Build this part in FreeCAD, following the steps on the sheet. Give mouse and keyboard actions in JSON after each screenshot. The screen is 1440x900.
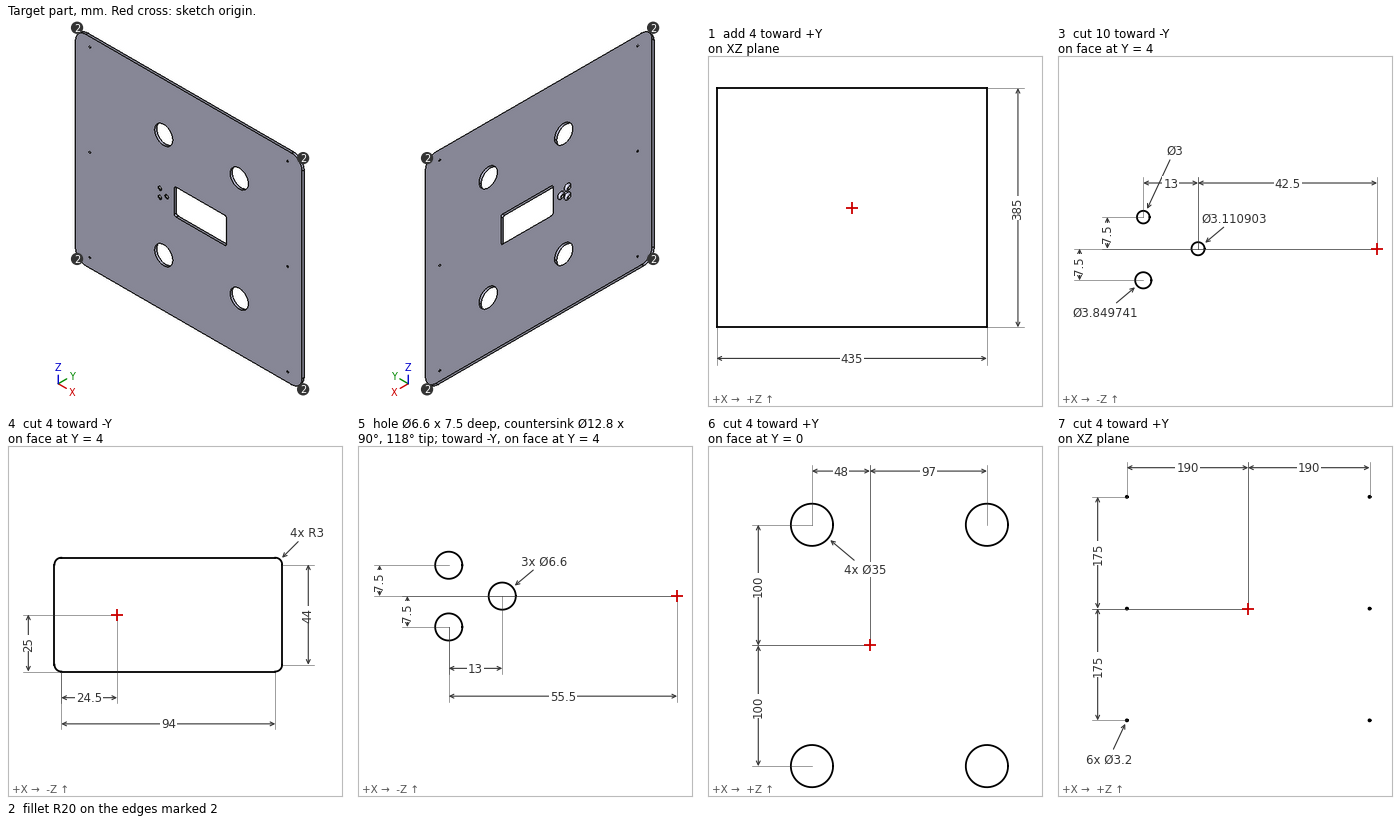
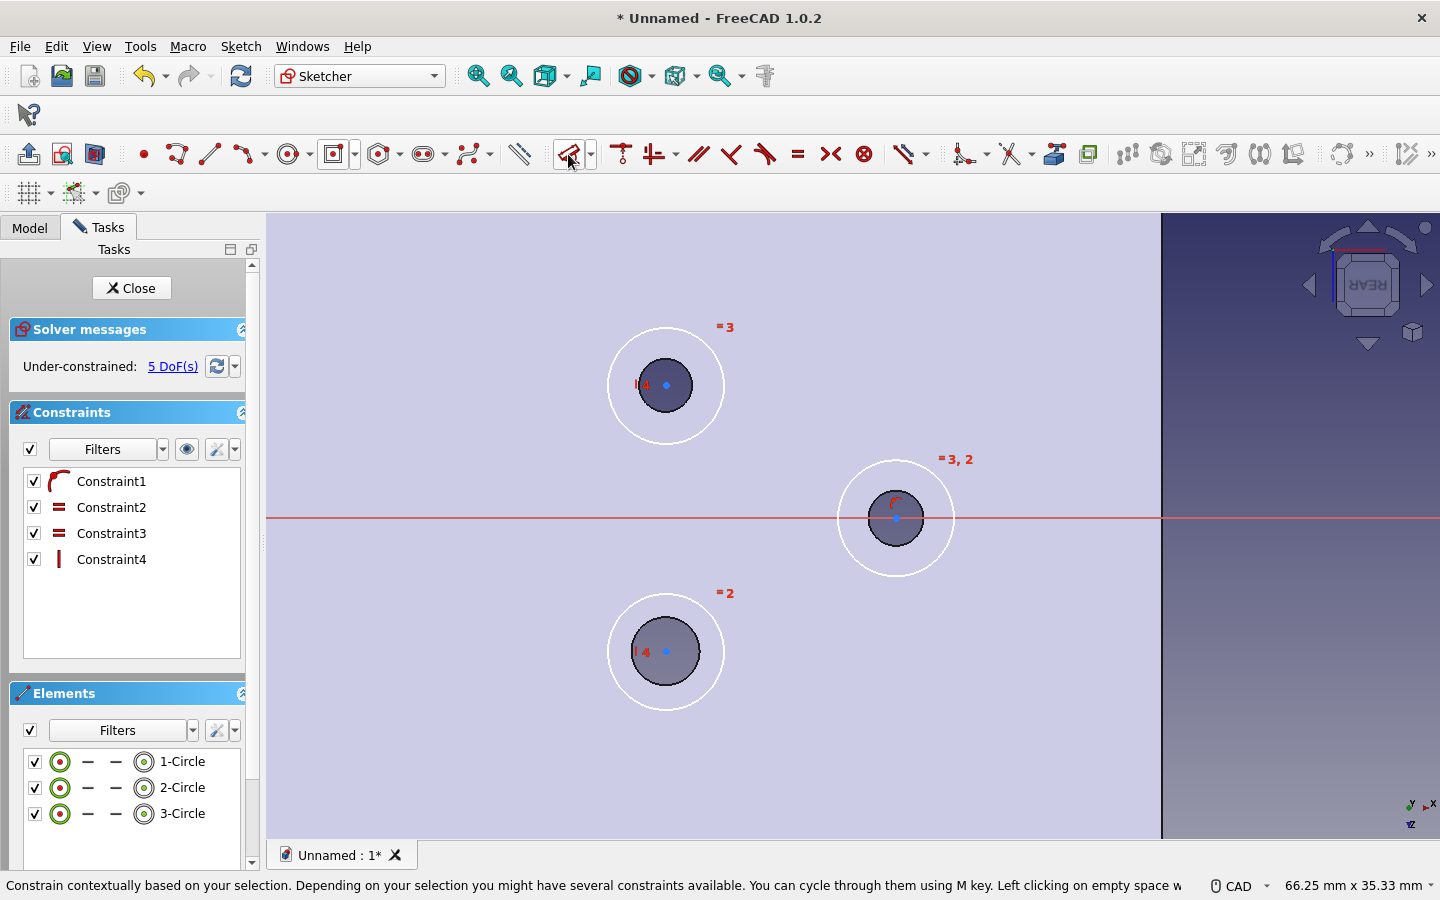
{"action": "left_click", "coordinate": [707, 611]}
{"action": "left_click", "coordinate": [730, 588]}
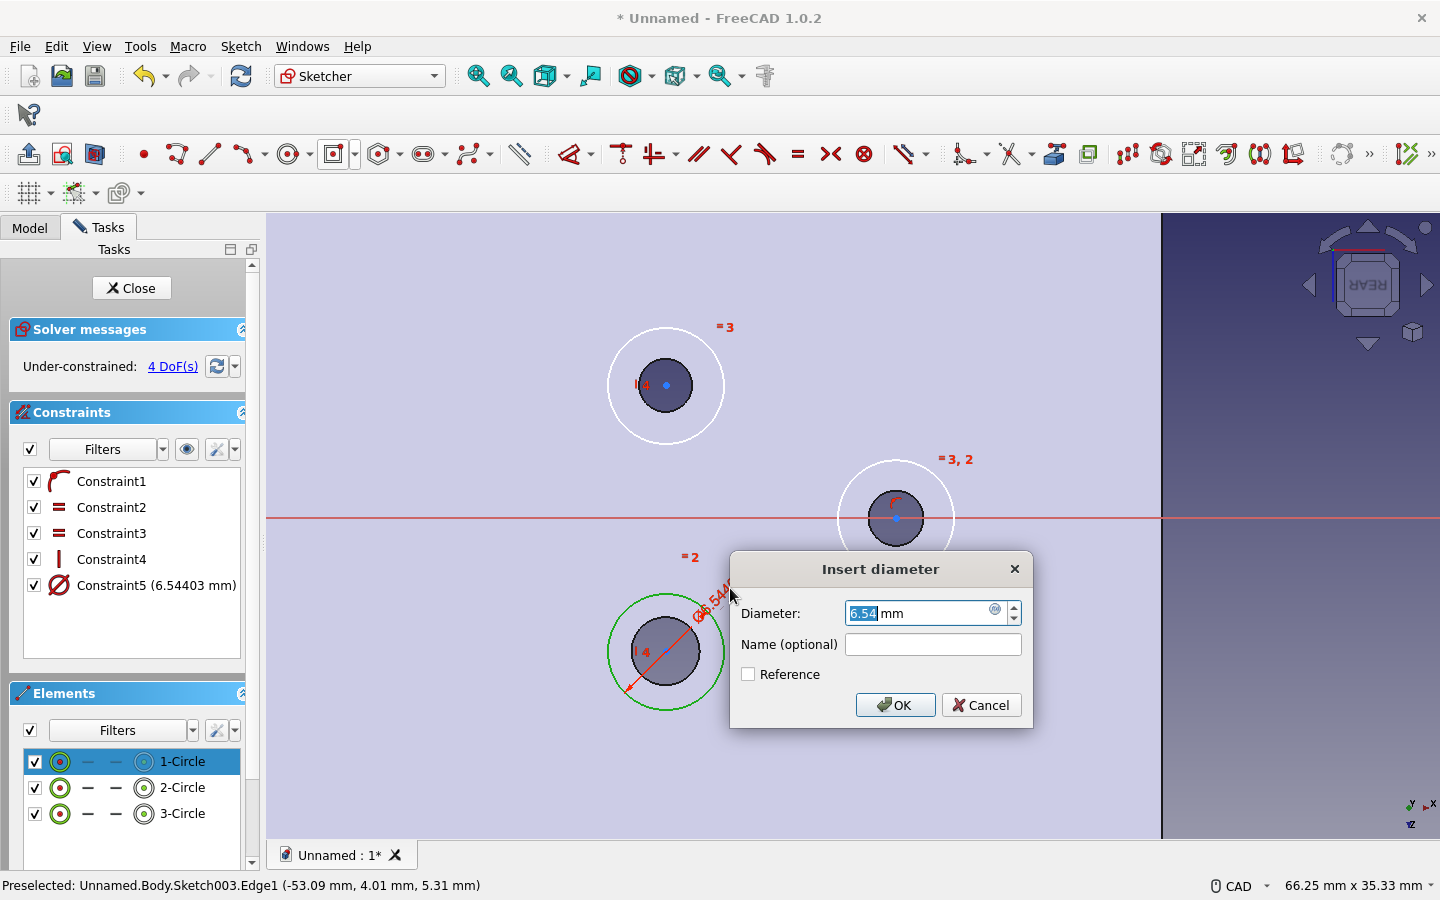
{"action": "type", "text": "6.6"}
{"action": "key", "text": "Return"}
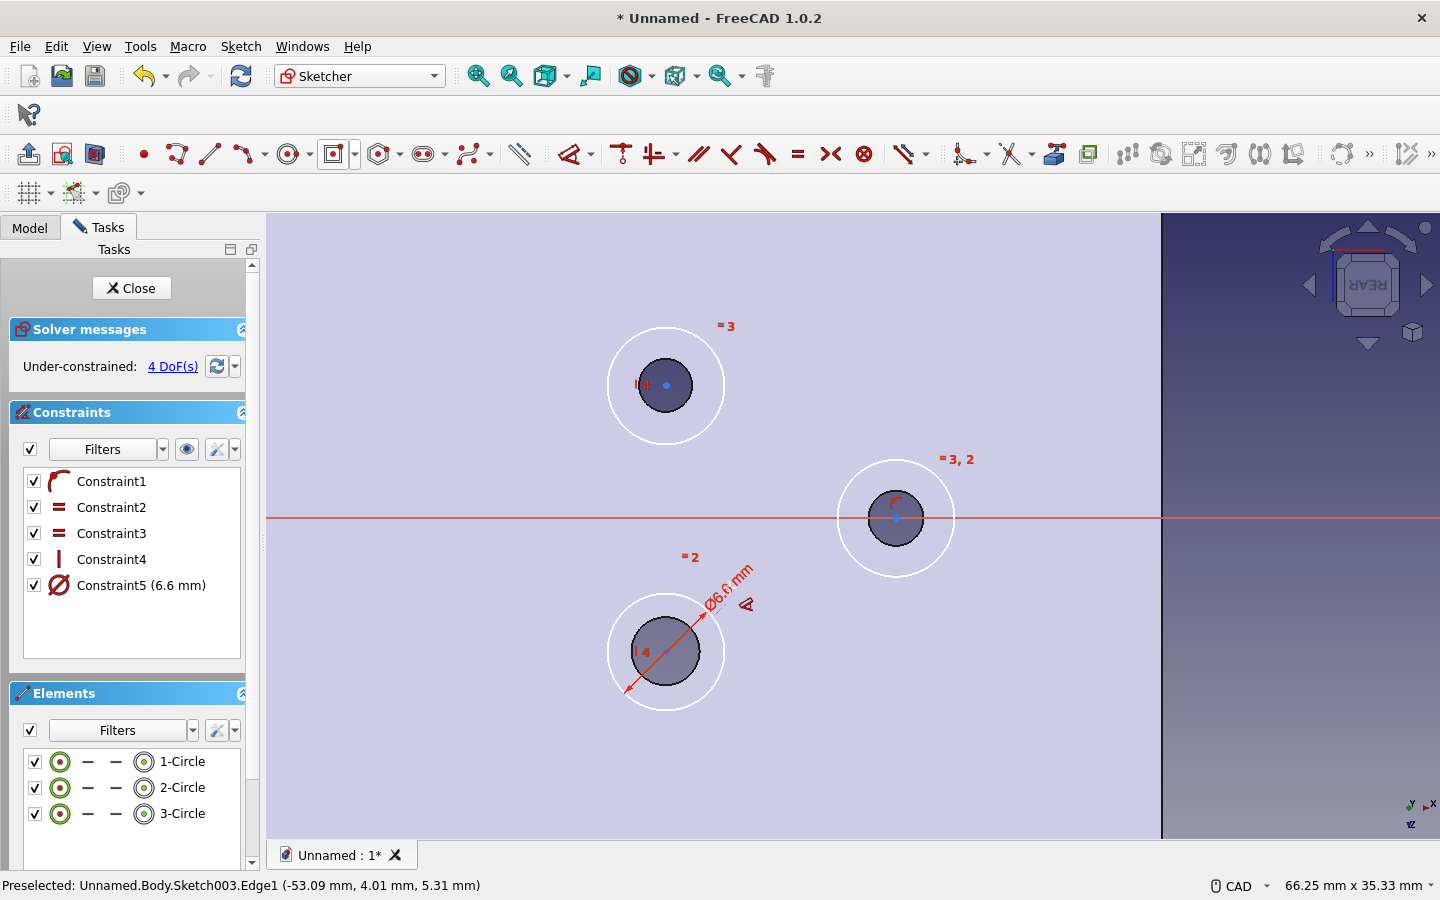
{"action": "left_click", "coordinate": [666, 652]}
{"action": "left_click", "coordinate": [632, 585]}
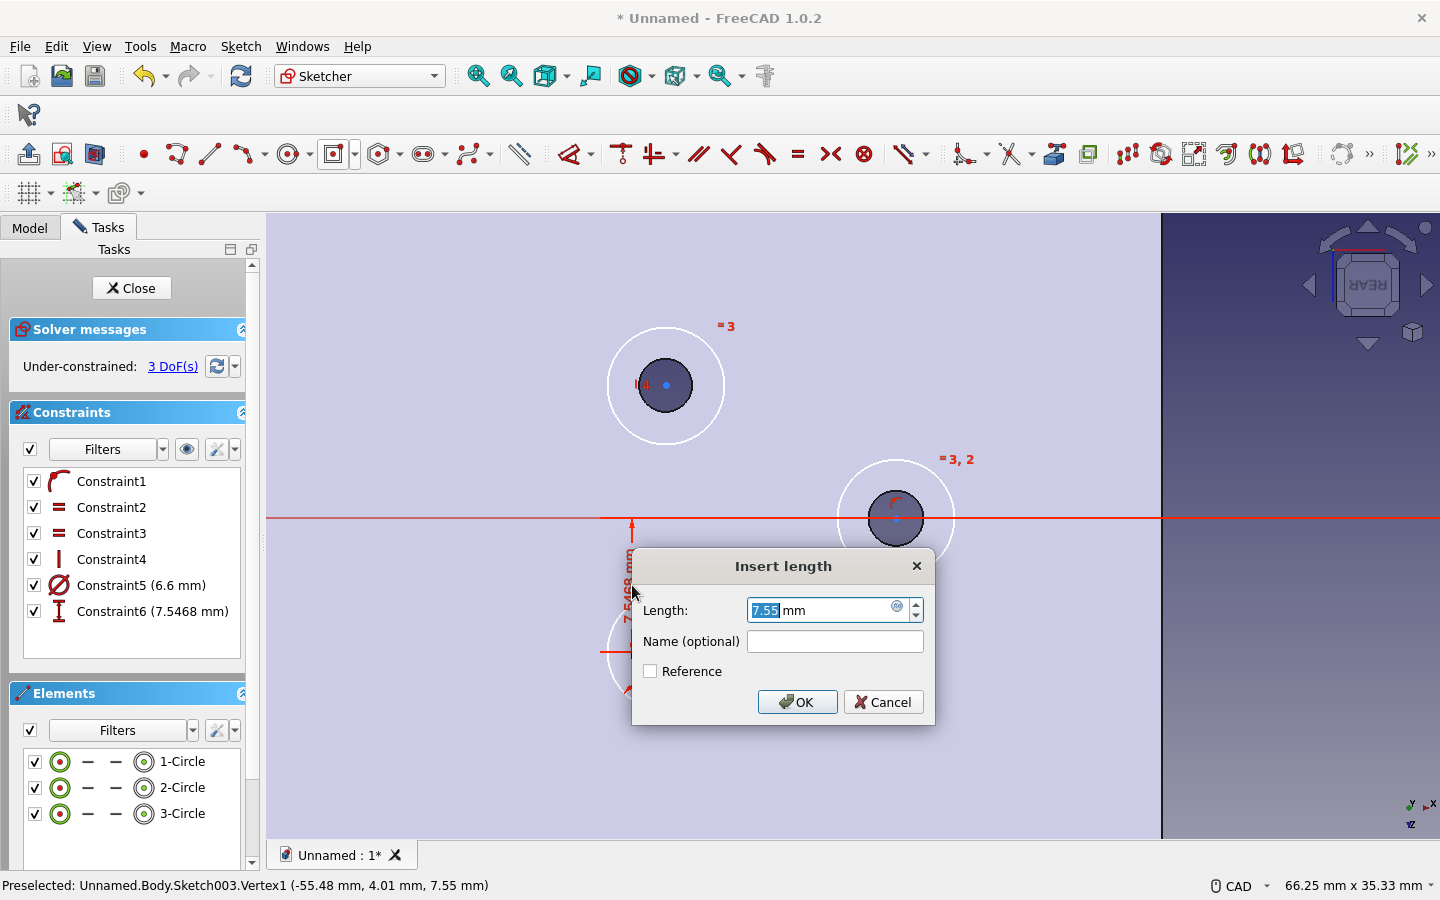
{"action": "type", "text": "7.5"}
{"action": "key", "text": "Return"}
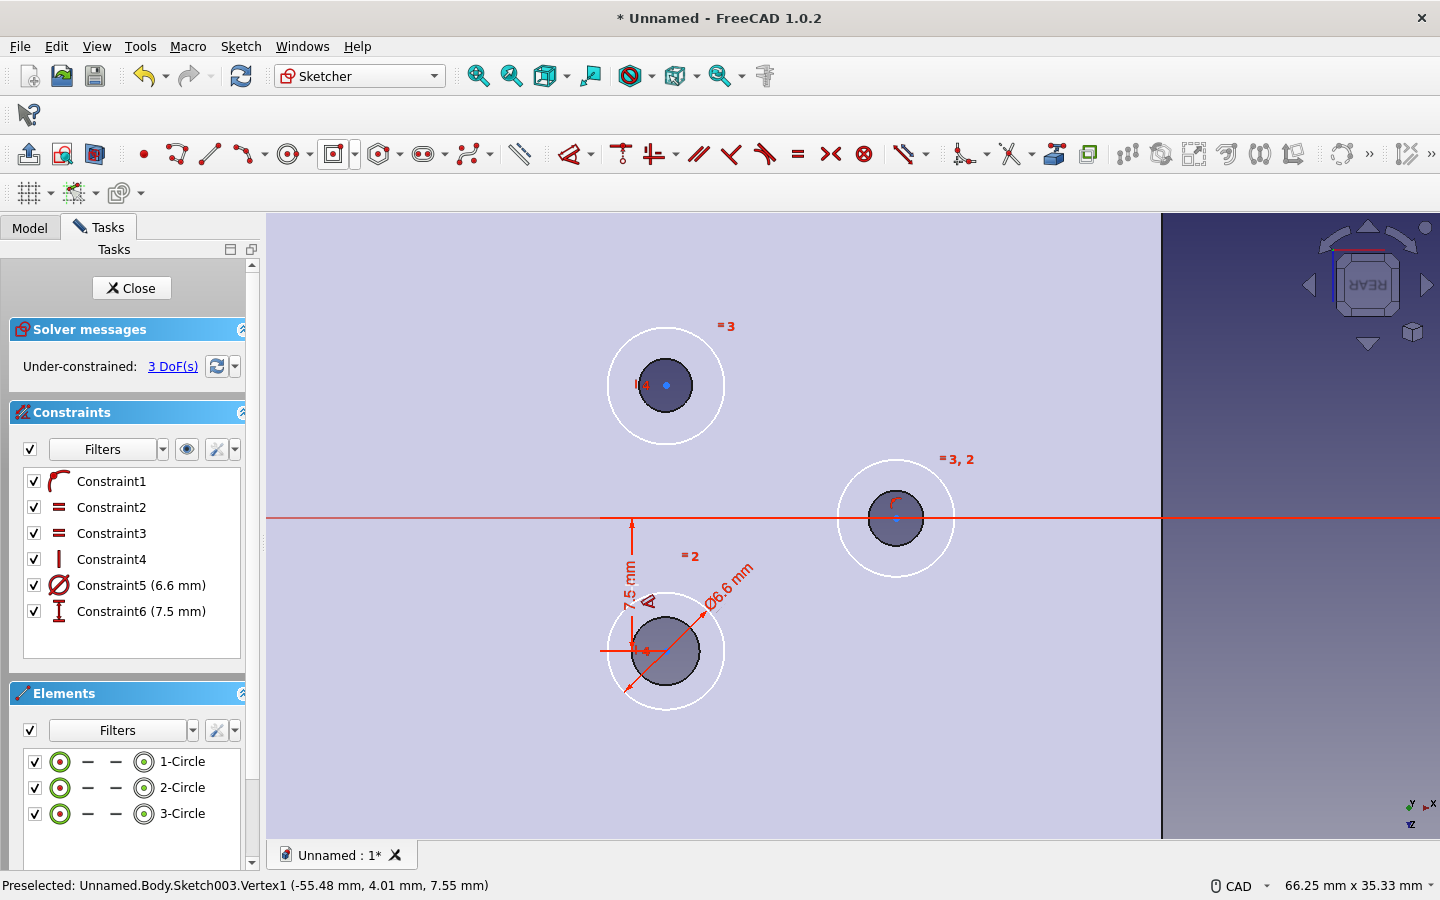
{"action": "left_click", "coordinate": [666, 386]}
{"action": "left_click", "coordinate": [632, 452]}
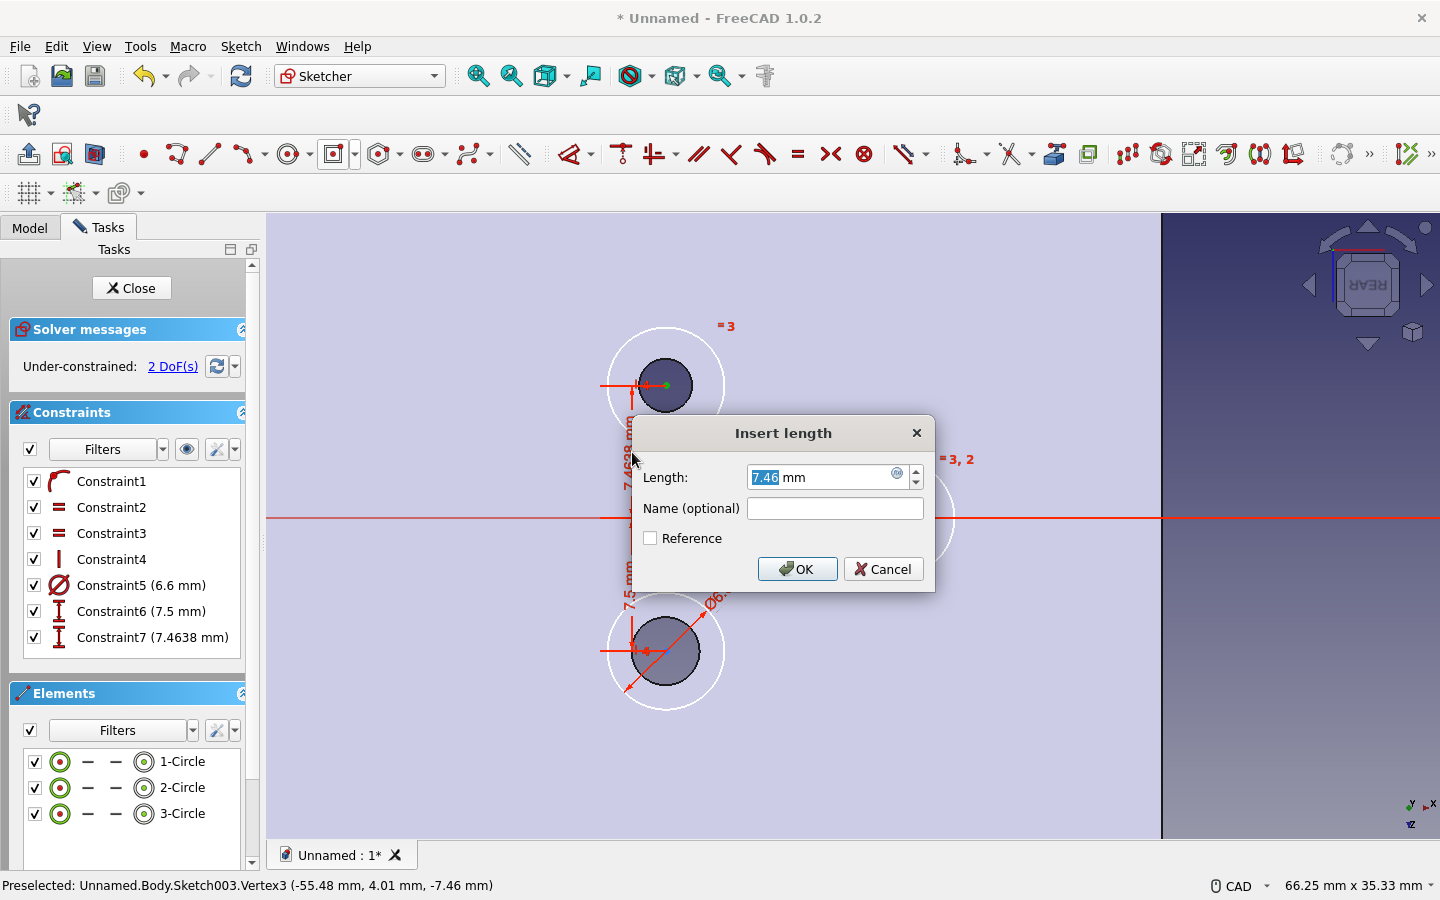
{"action": "type", "text": "7.5"}
{"action": "key", "text": "Return"}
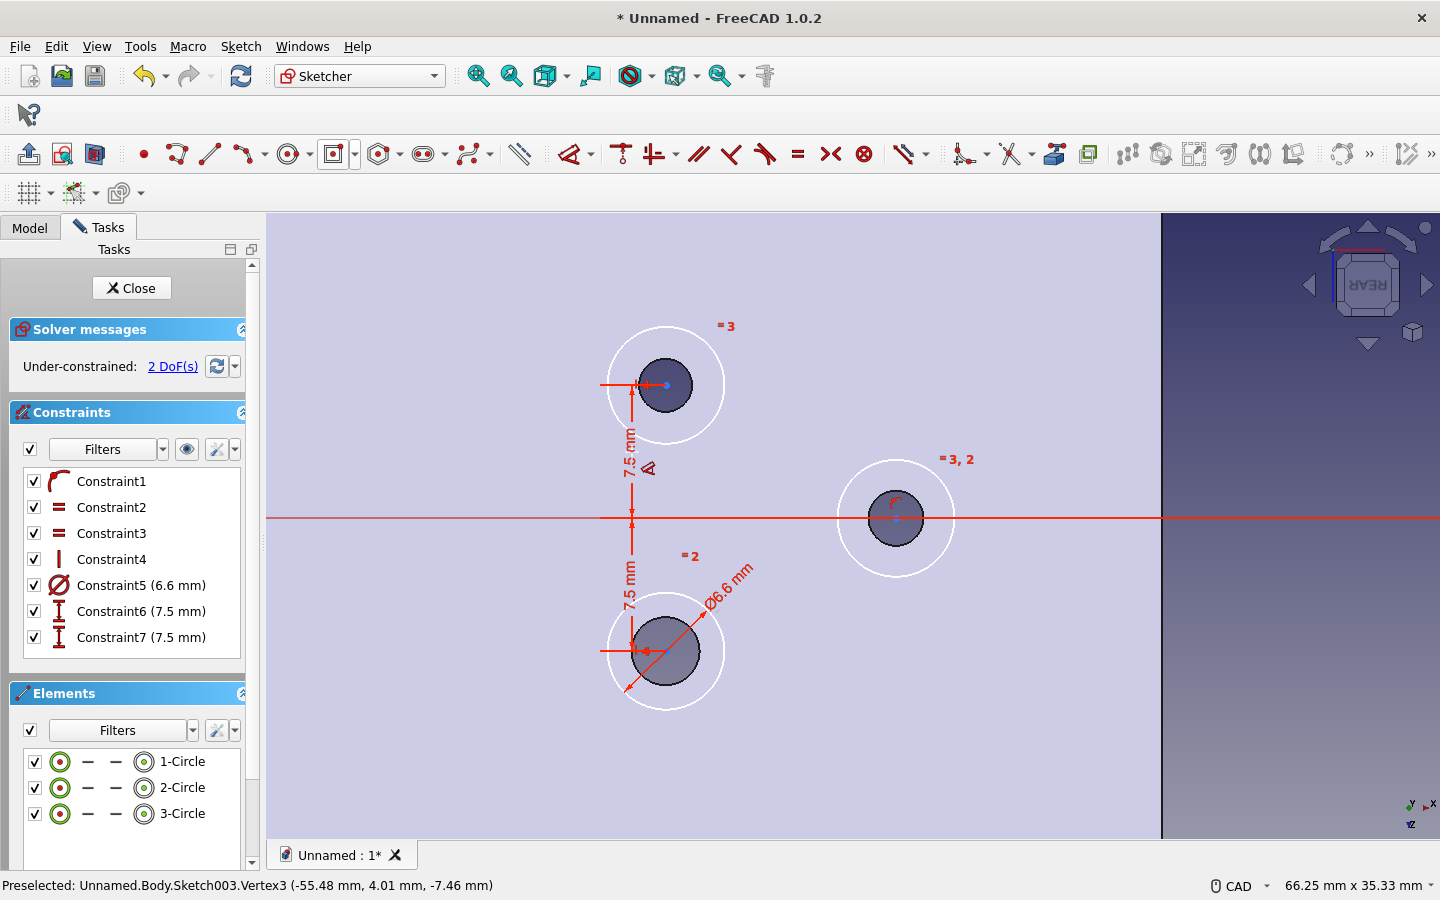
{"action": "left_click", "coordinate": [666, 651]}